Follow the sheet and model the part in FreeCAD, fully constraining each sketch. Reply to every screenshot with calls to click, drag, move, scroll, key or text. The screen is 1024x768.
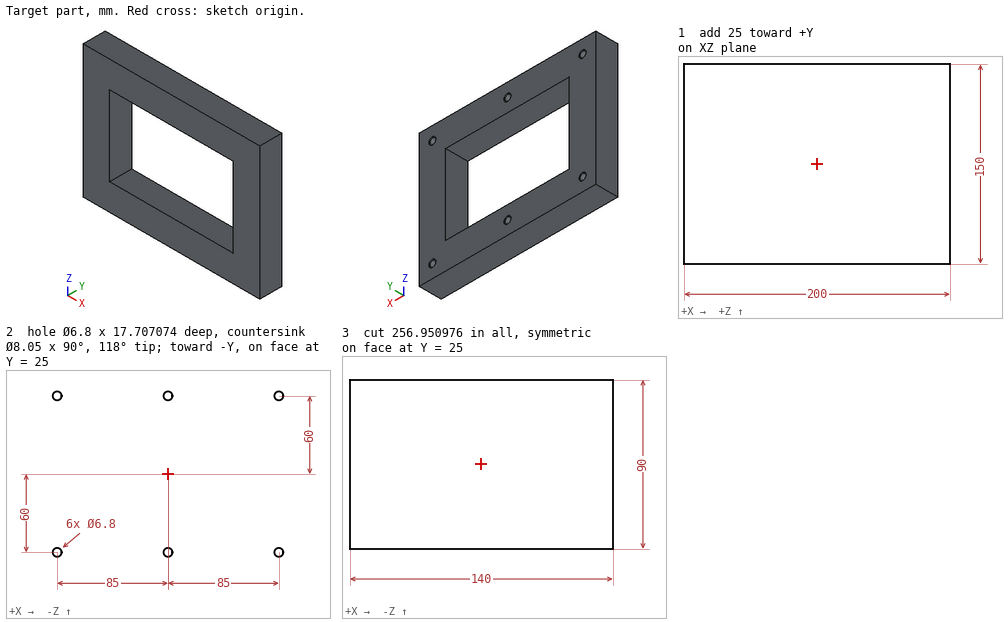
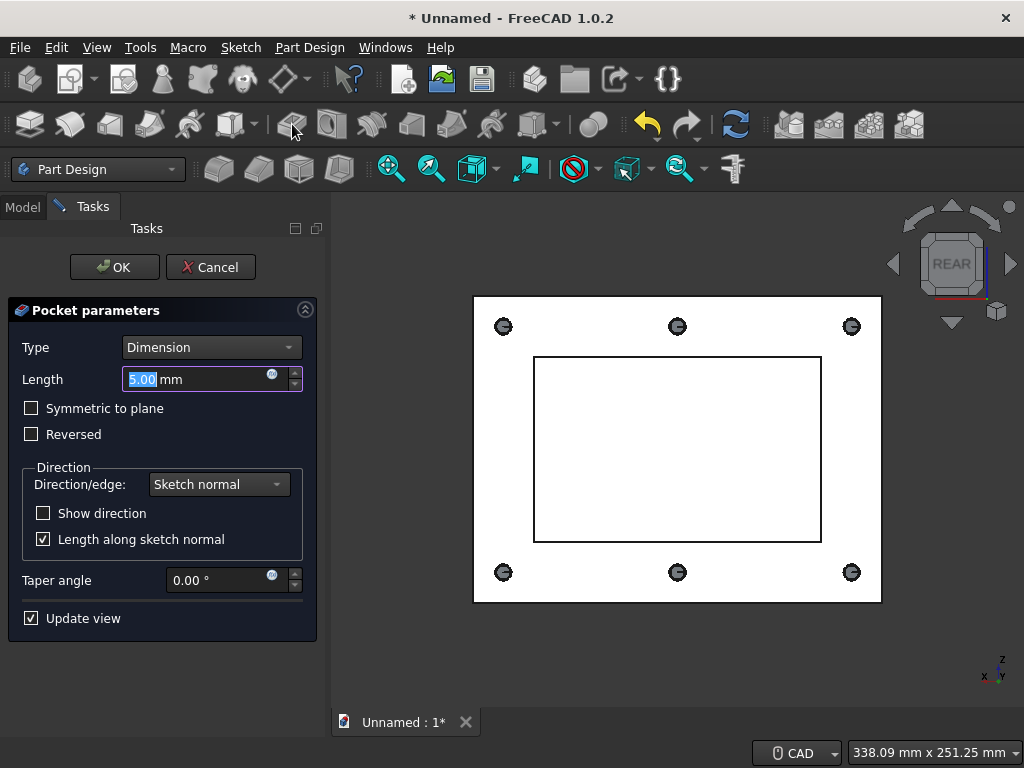
text(256.950976)
key(Tab)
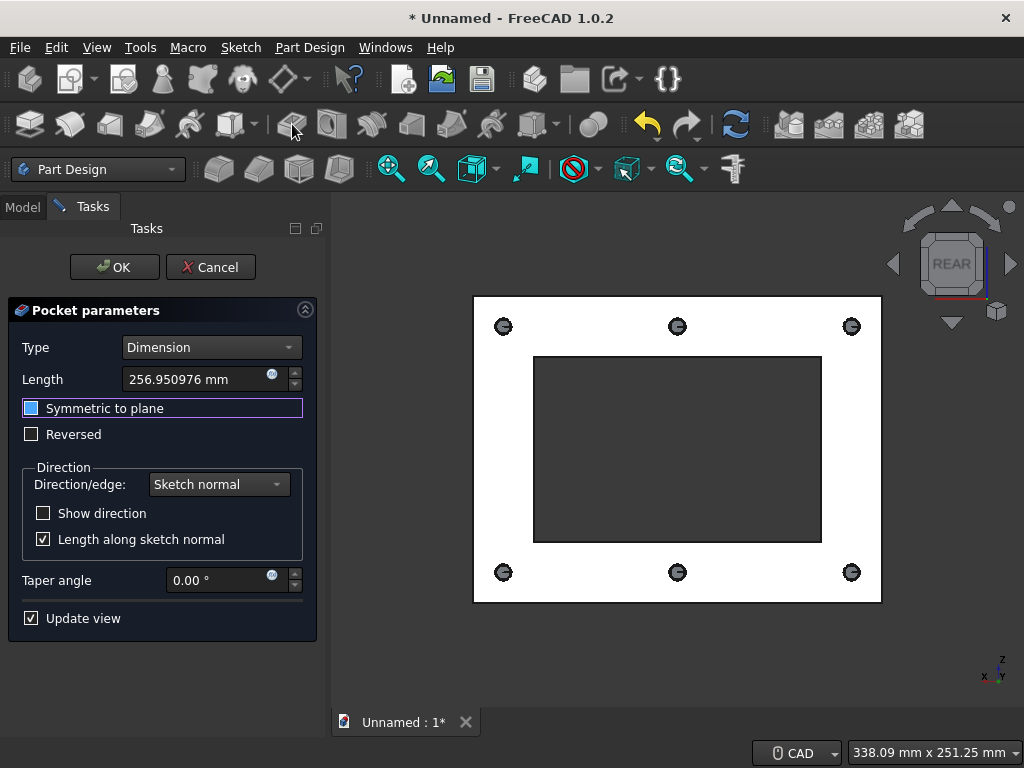
click(30, 408)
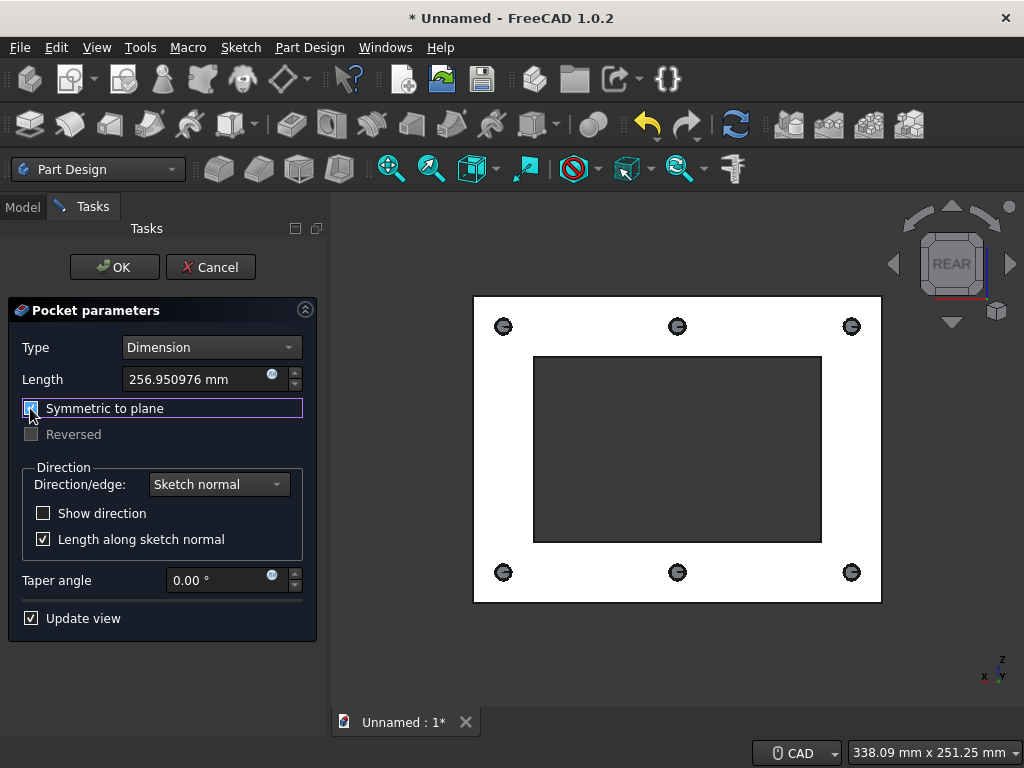
click(115, 267)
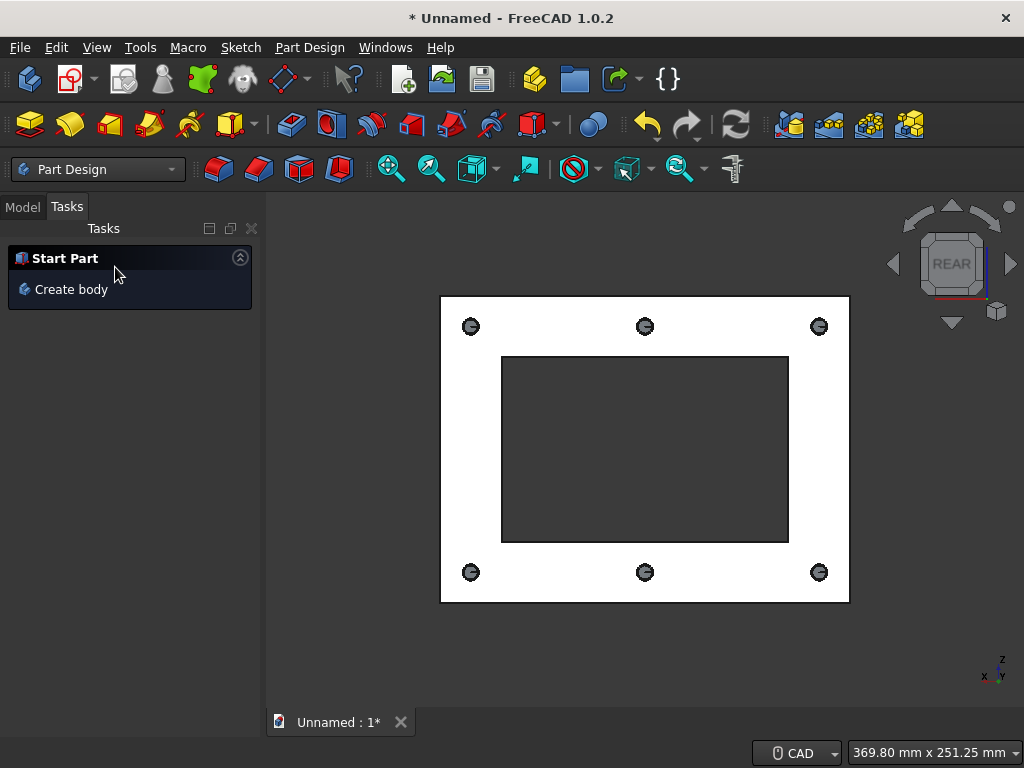
key(0)